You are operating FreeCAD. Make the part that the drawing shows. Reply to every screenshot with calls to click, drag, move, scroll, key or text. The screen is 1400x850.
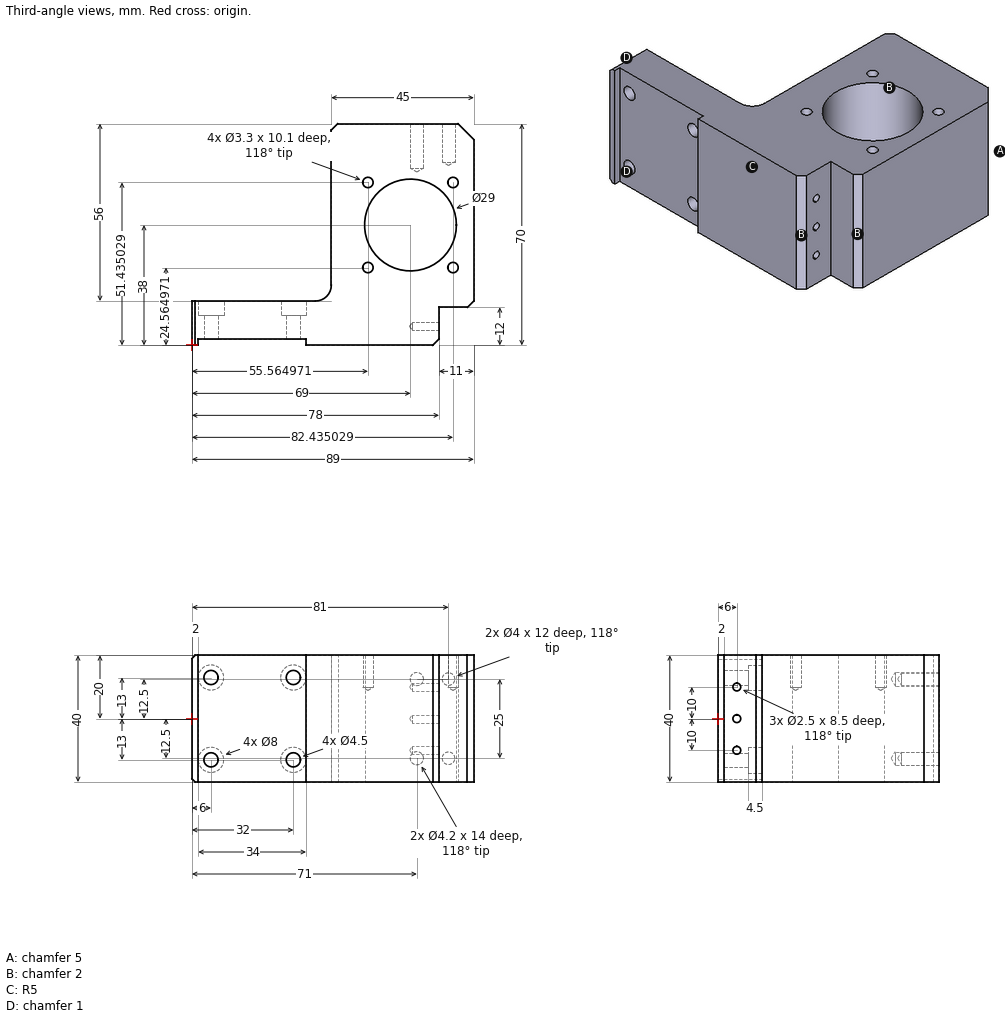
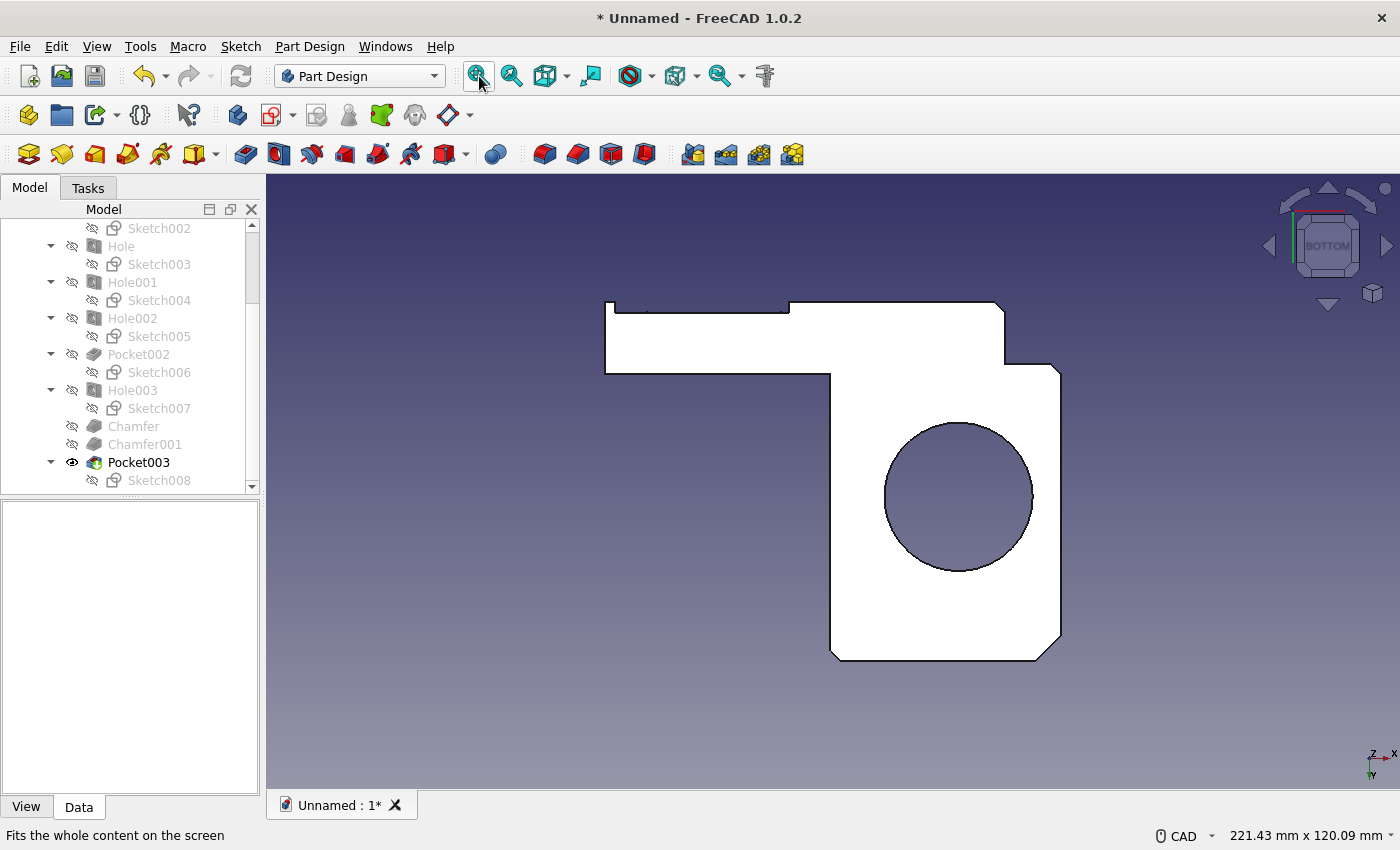
key(4)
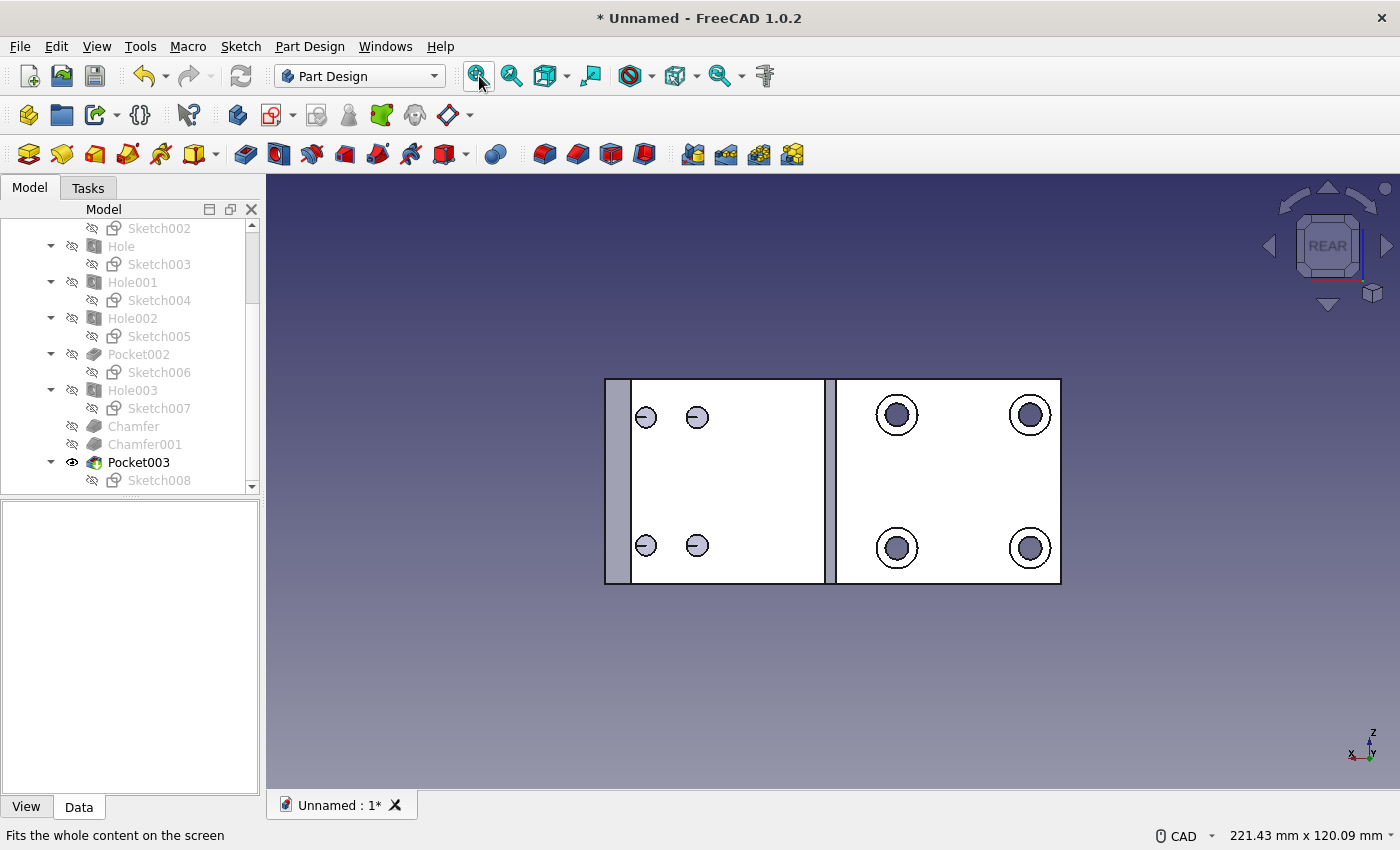
click(479, 76)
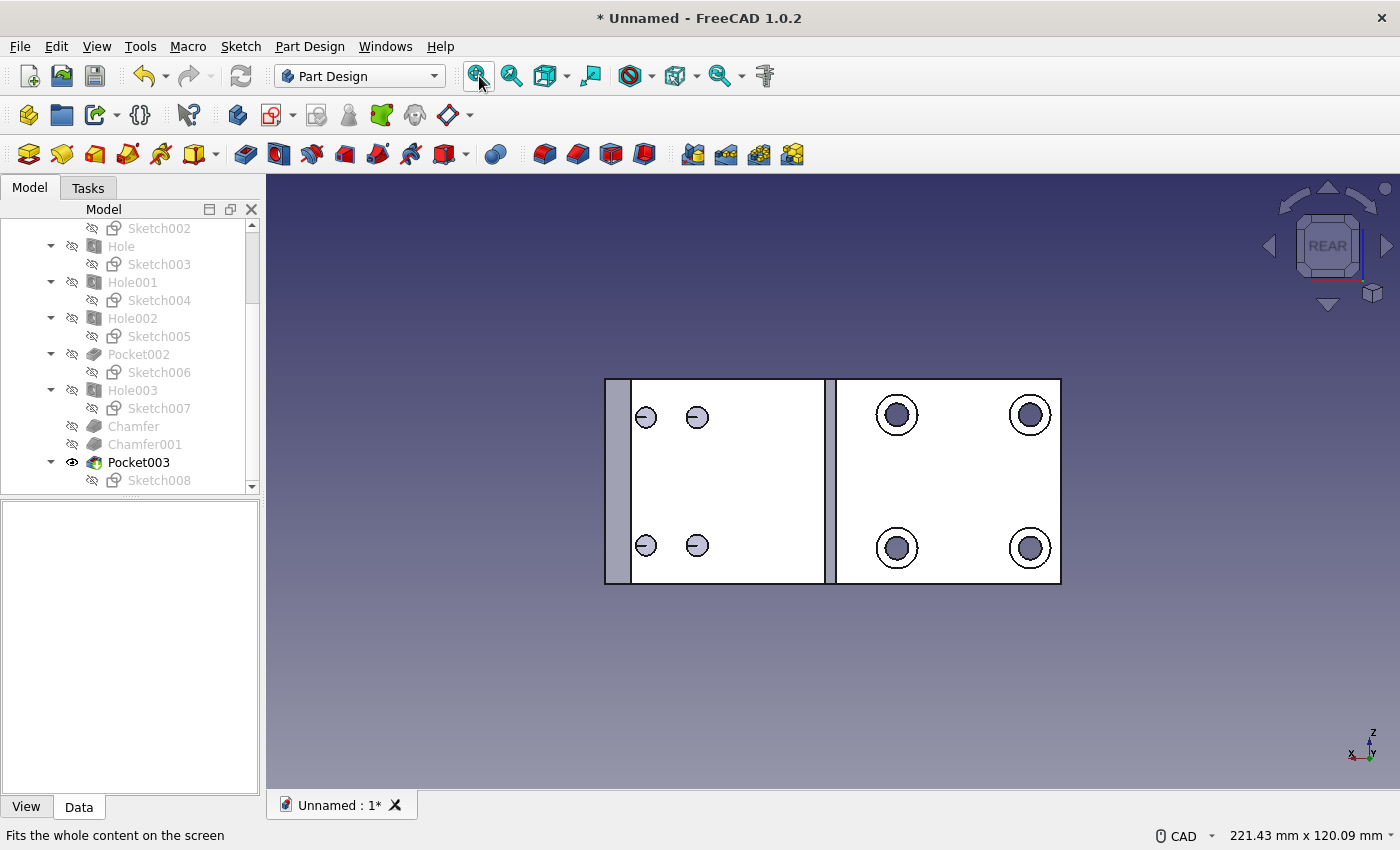
key(6)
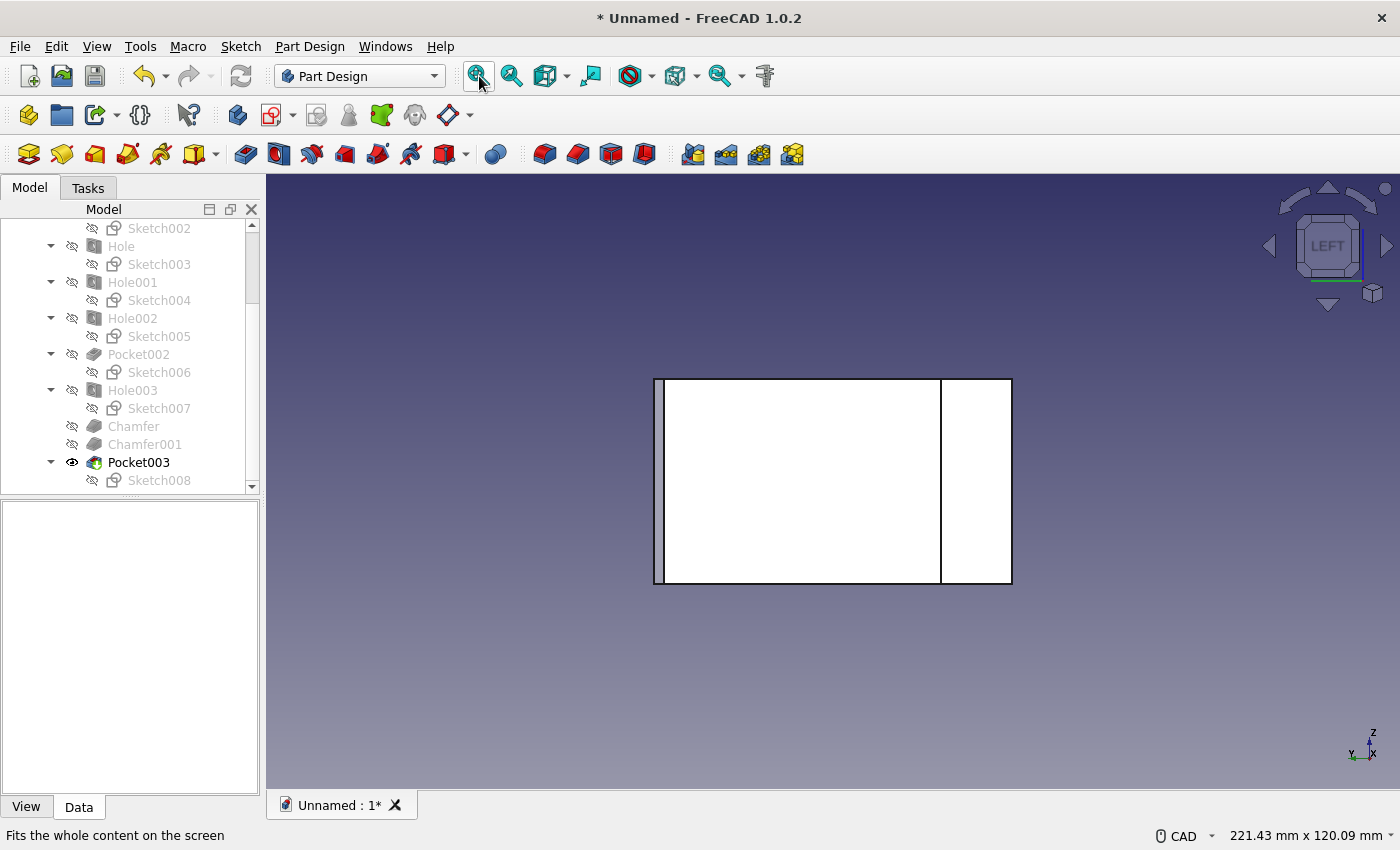
key(v)
key(f)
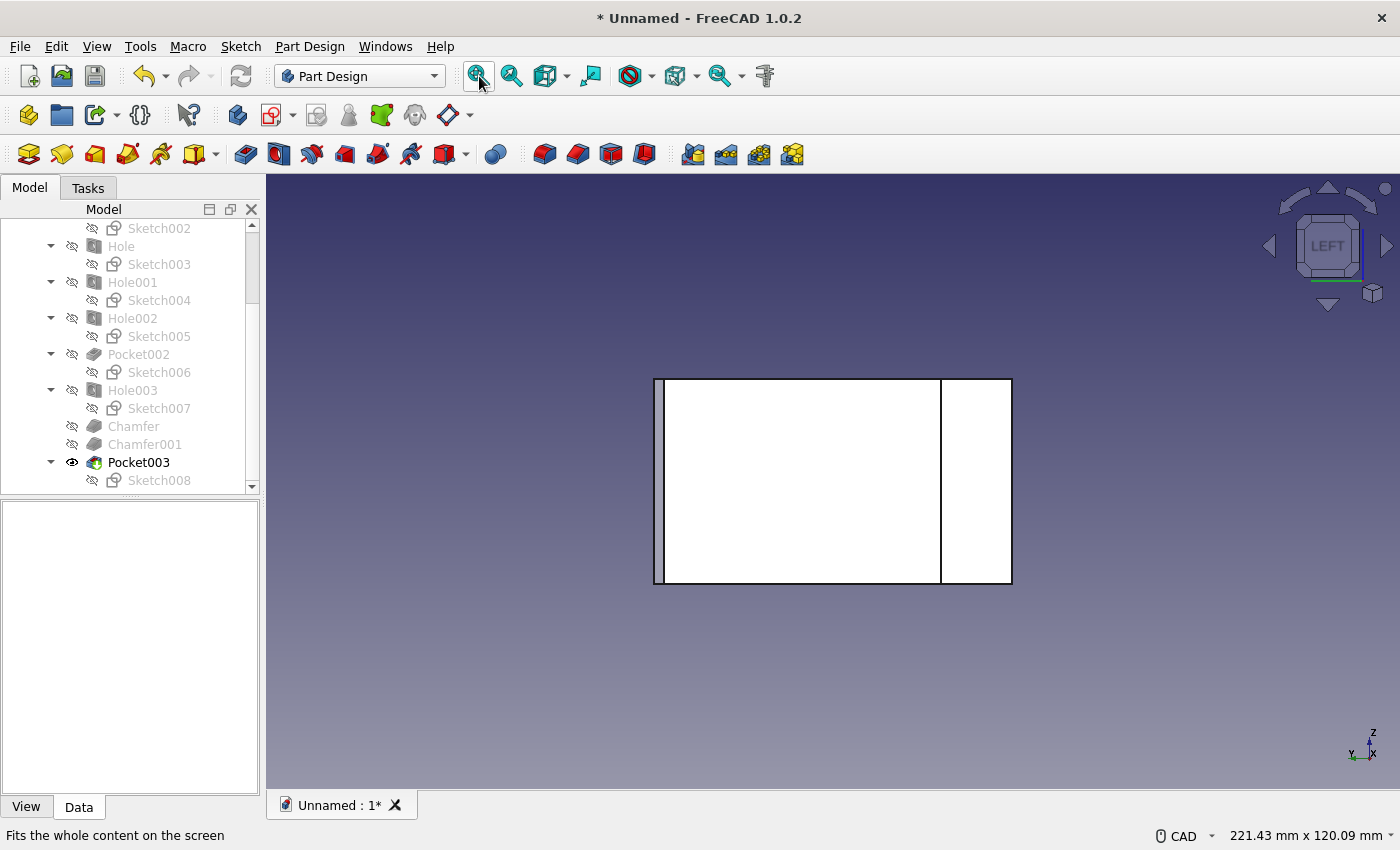
key(v)
key(3)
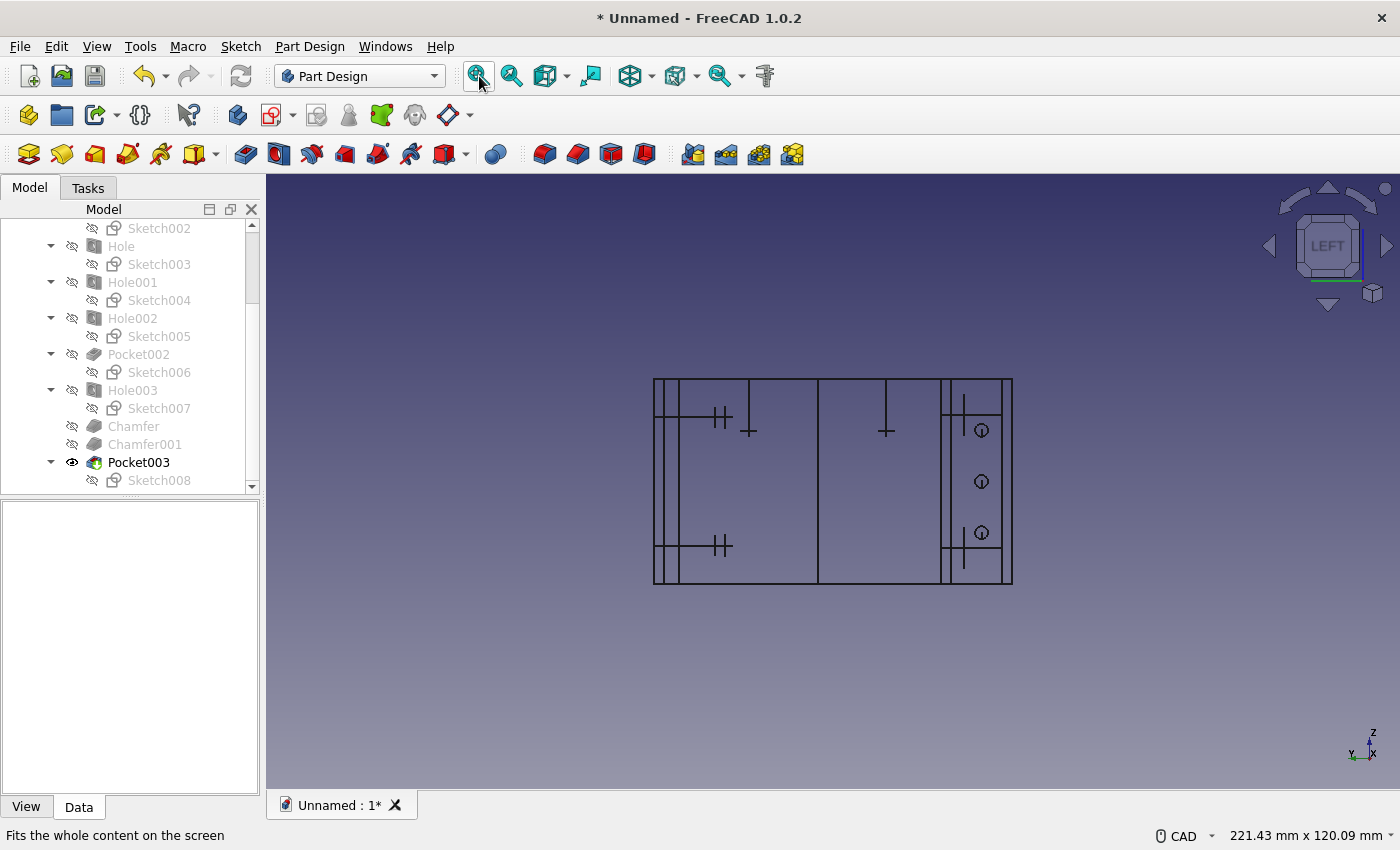
key(0)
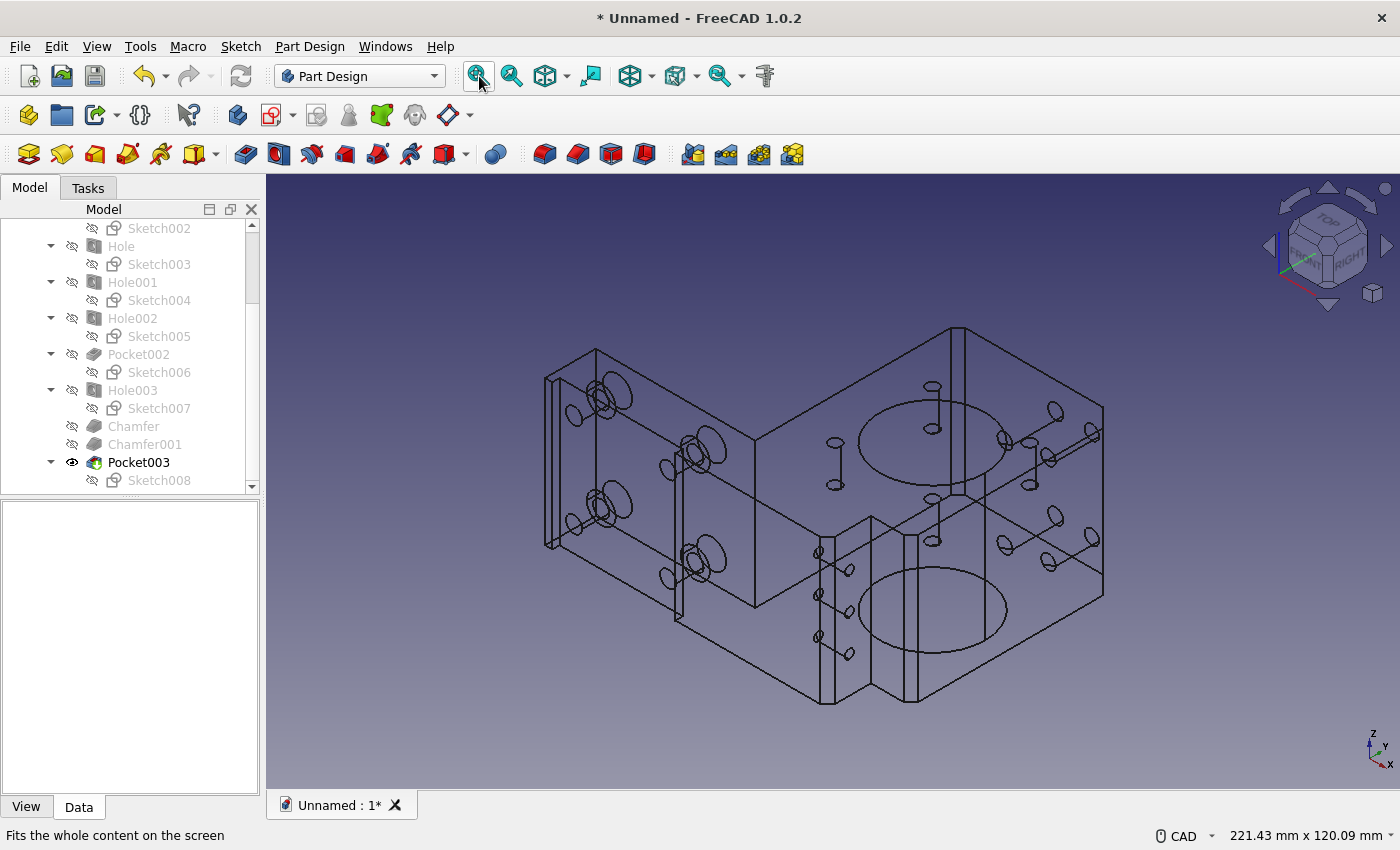
click(755, 523)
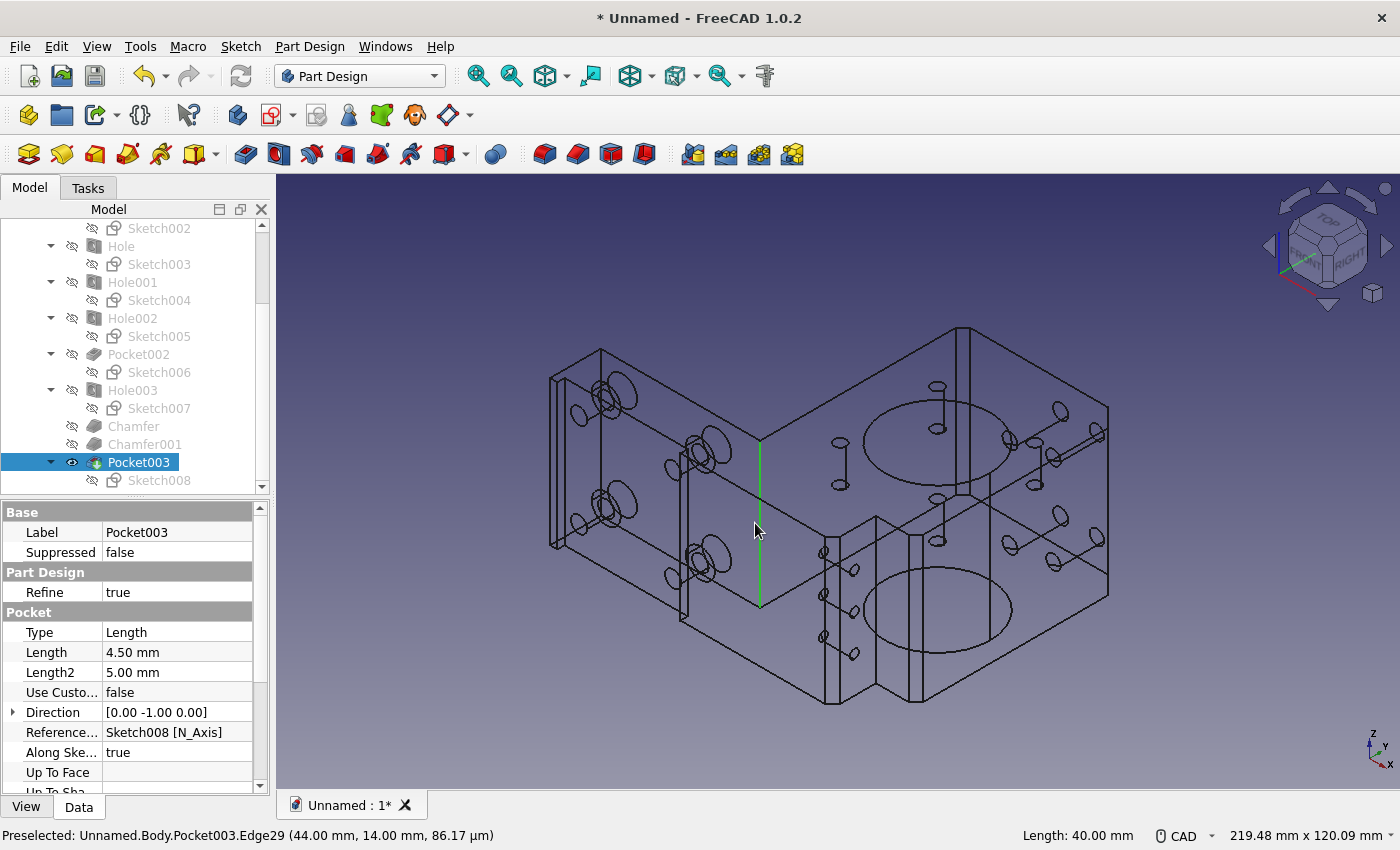
key(v)
key(1)